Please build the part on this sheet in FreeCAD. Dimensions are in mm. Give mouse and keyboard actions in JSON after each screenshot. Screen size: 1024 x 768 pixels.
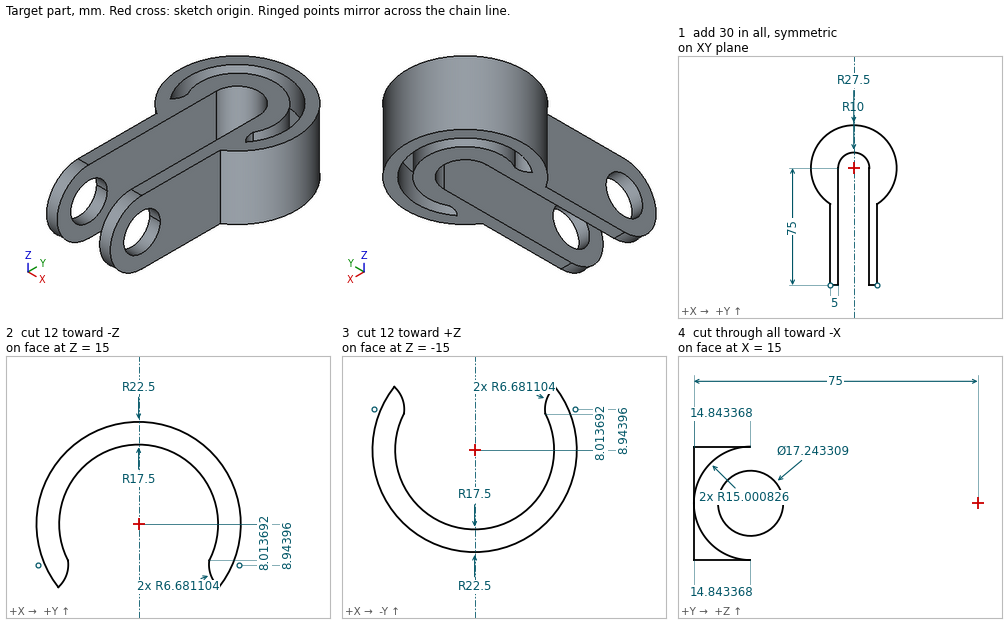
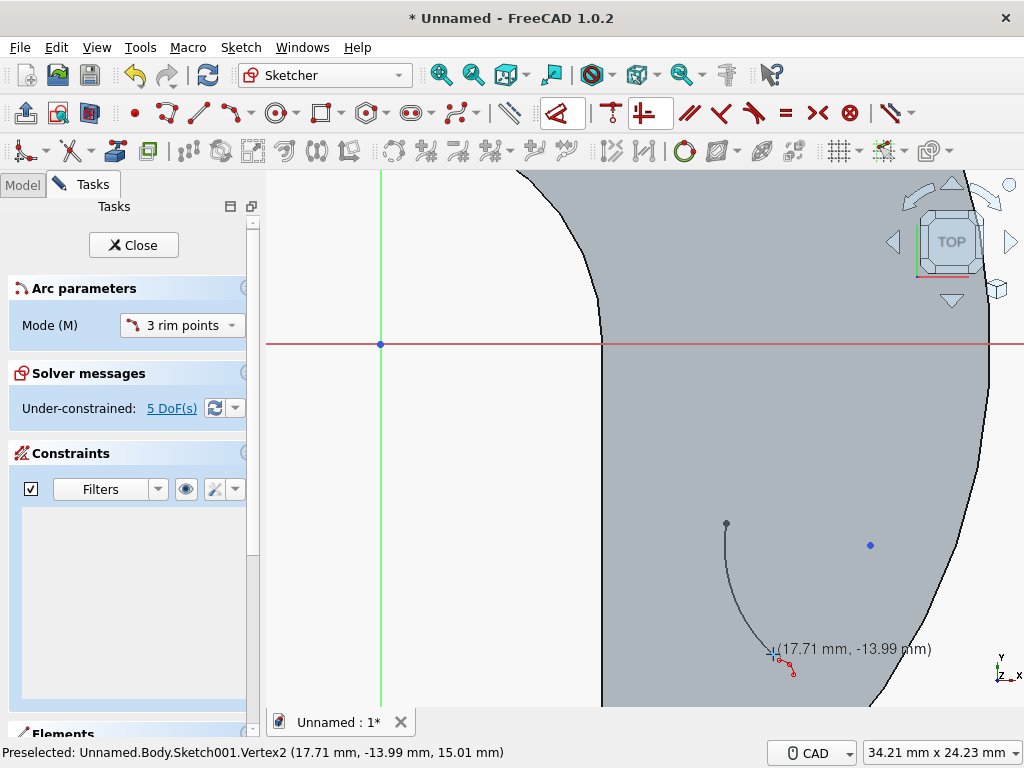
{"action": "scroll", "coordinate": [736, 593], "scroll_direction": "down", "scroll_amount": 4}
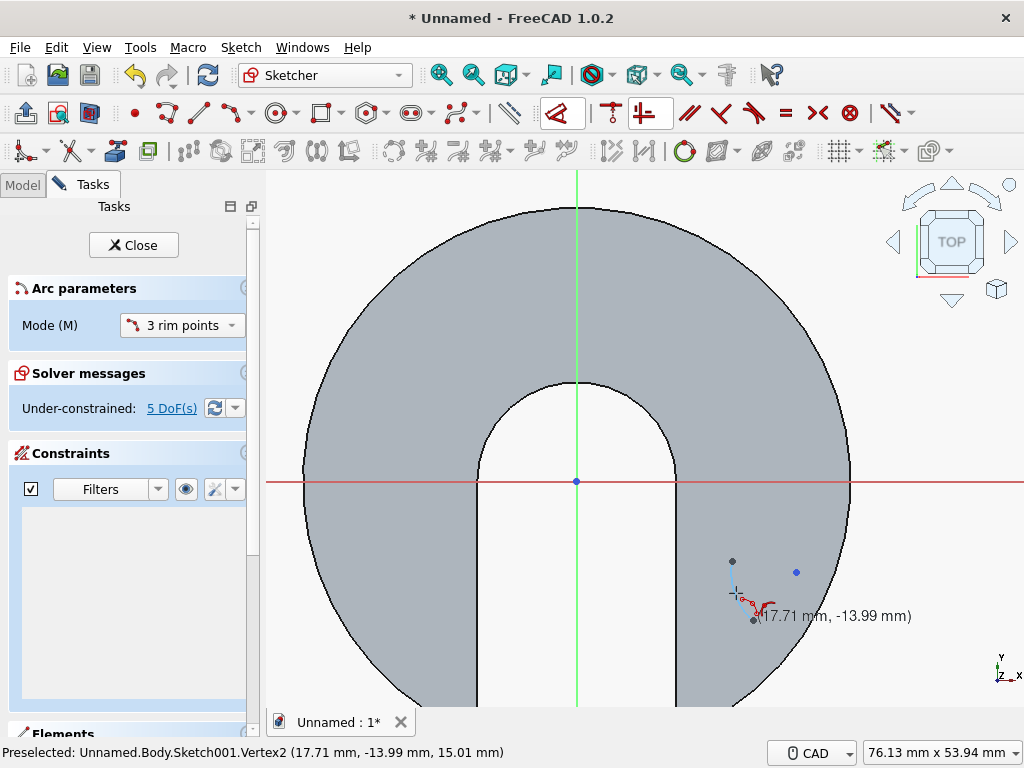
{"action": "left_click", "coordinate": [401, 620]}
{"action": "left_click", "coordinate": [674, 280]}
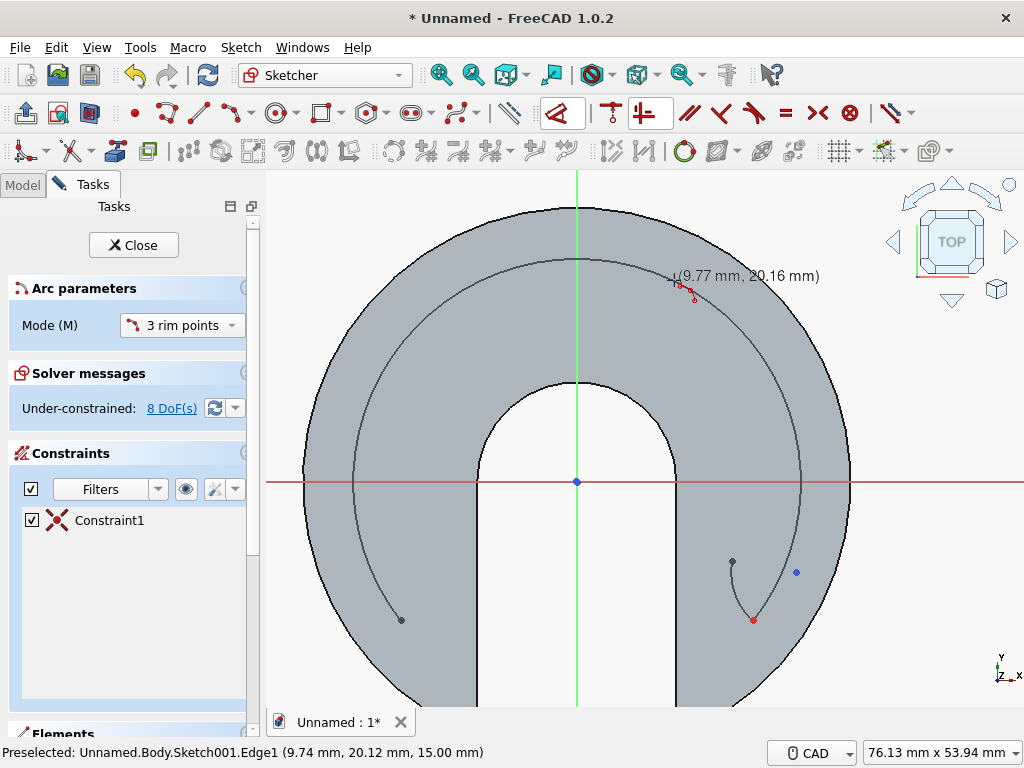
{"action": "left_click", "coordinate": [401, 621]}
{"action": "left_click", "coordinate": [422, 561]}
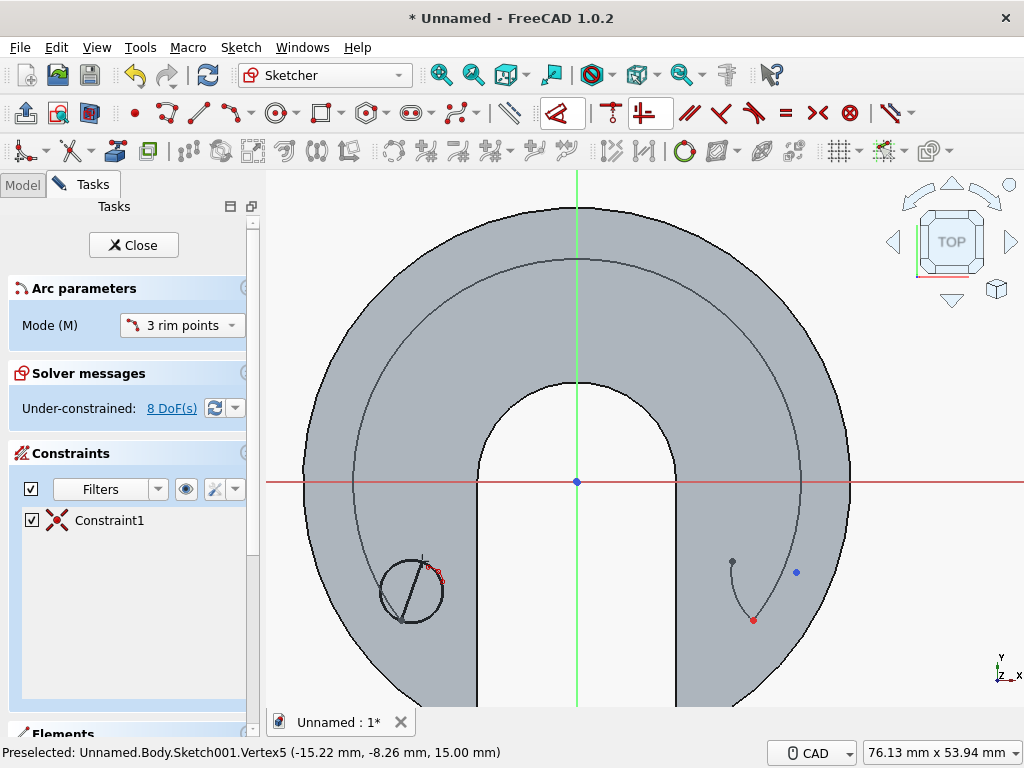
{"action": "scroll", "coordinate": [419, 593], "scroll_direction": "up", "scroll_amount": 4}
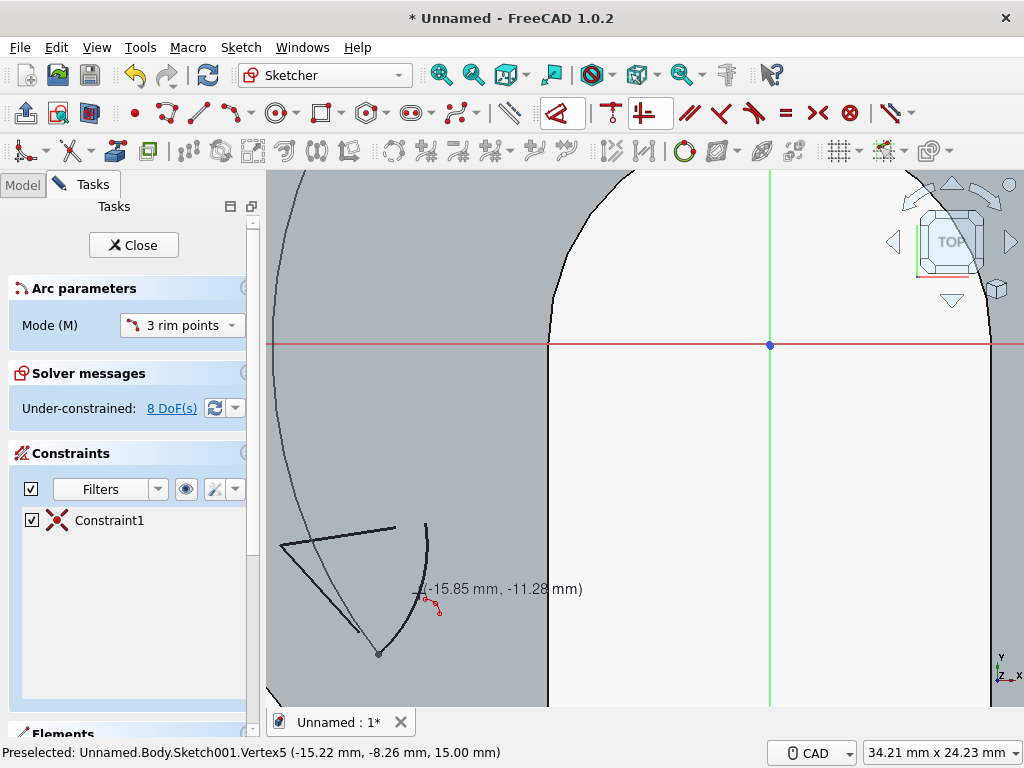
{"action": "left_click", "coordinate": [418, 593]}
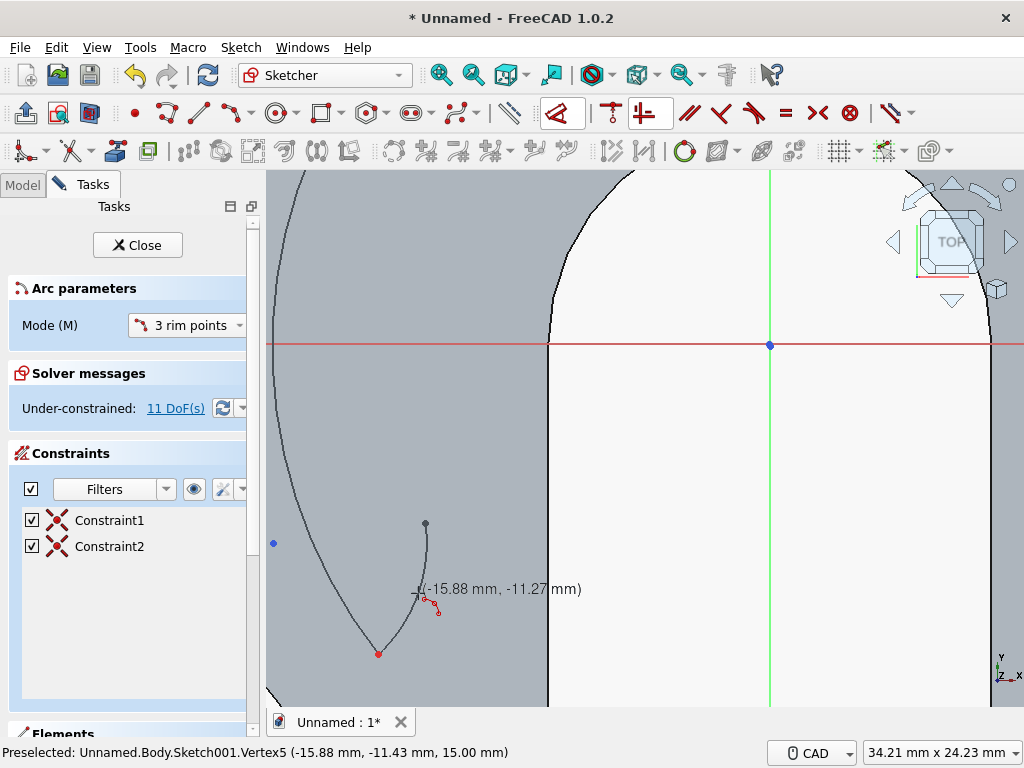
{"action": "left_click", "coordinate": [425, 523]}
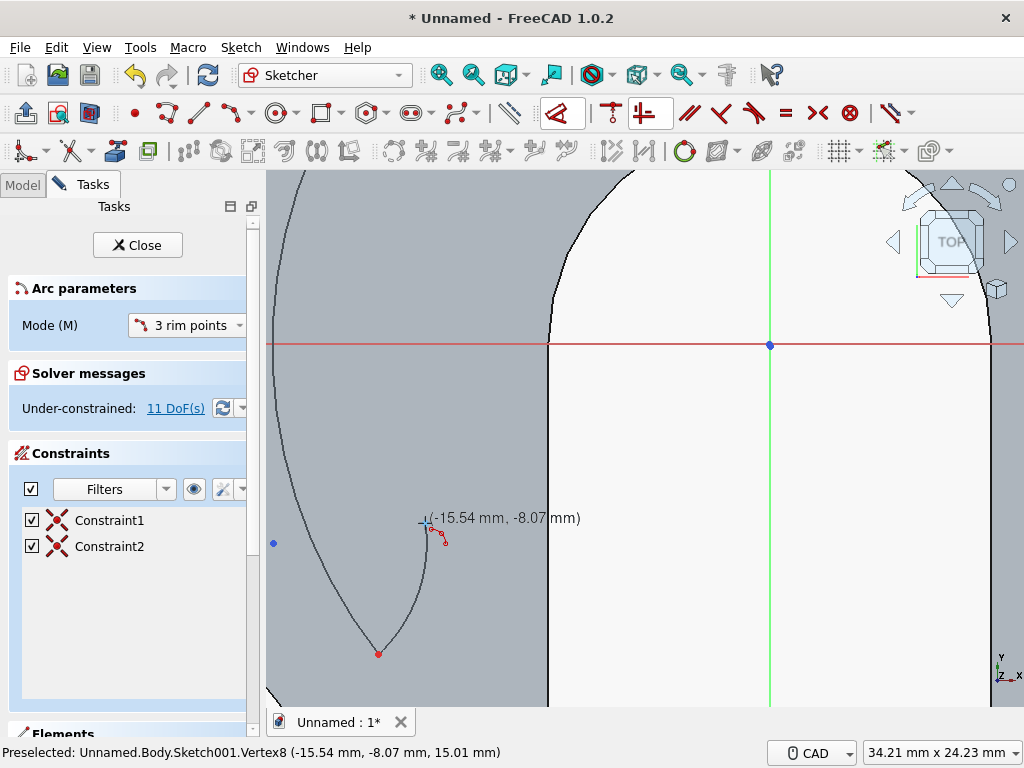
{"action": "scroll", "coordinate": [419, 593], "scroll_direction": "down", "scroll_amount": 4}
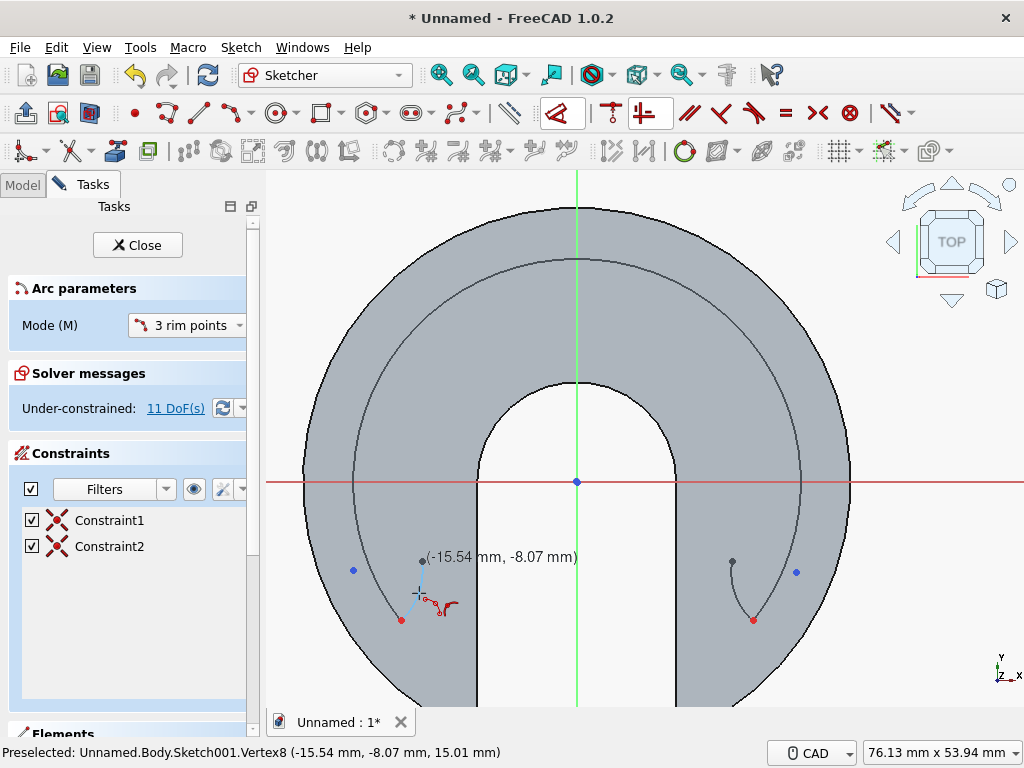
{"action": "left_click", "coordinate": [732, 562]}
{"action": "left_click", "coordinate": [646, 322]}
{"action": "key", "text": "Escape"}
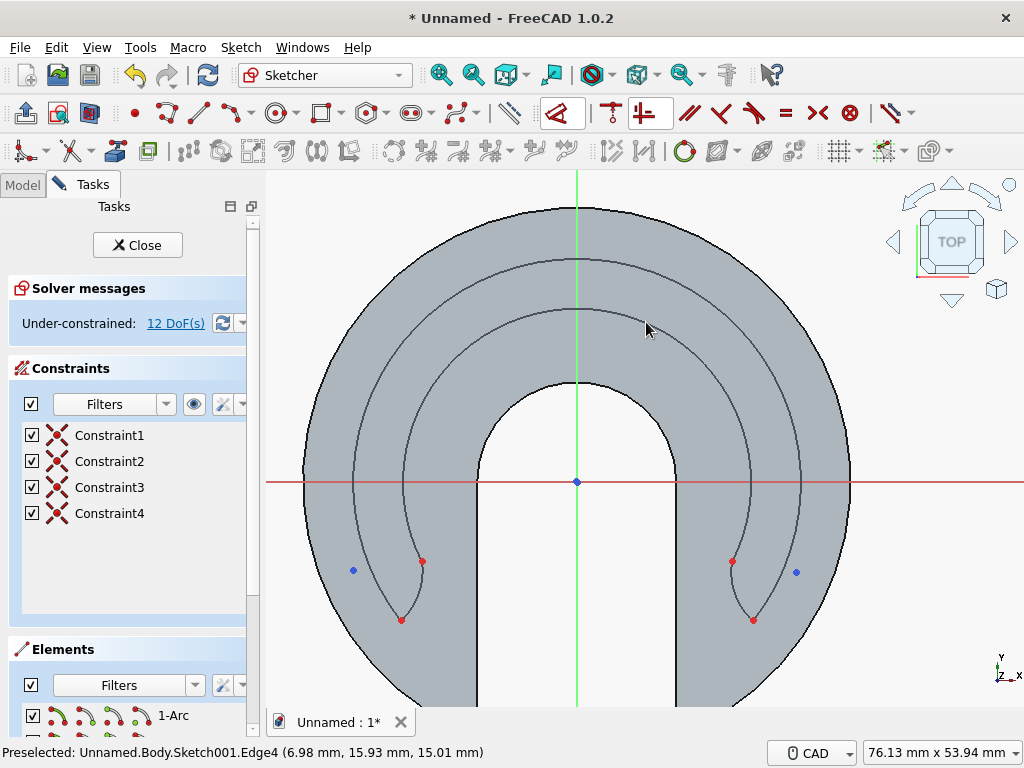
{"action": "left_click", "coordinate": [752, 343]}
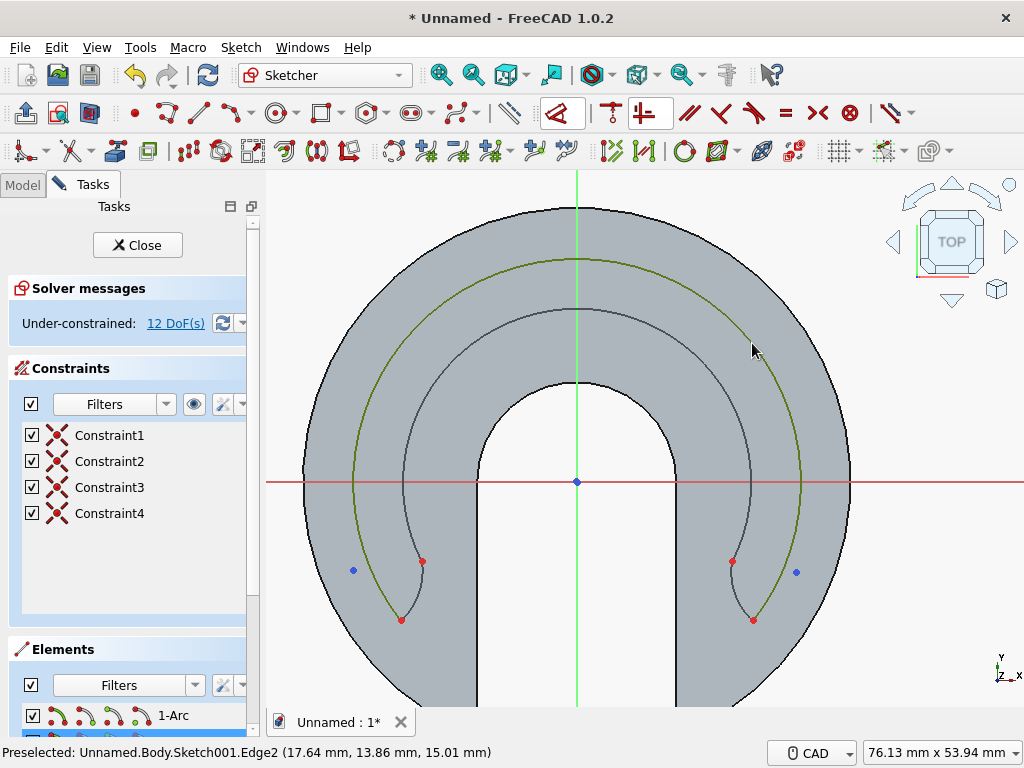
{"action": "left_click", "coordinate": [704, 364]}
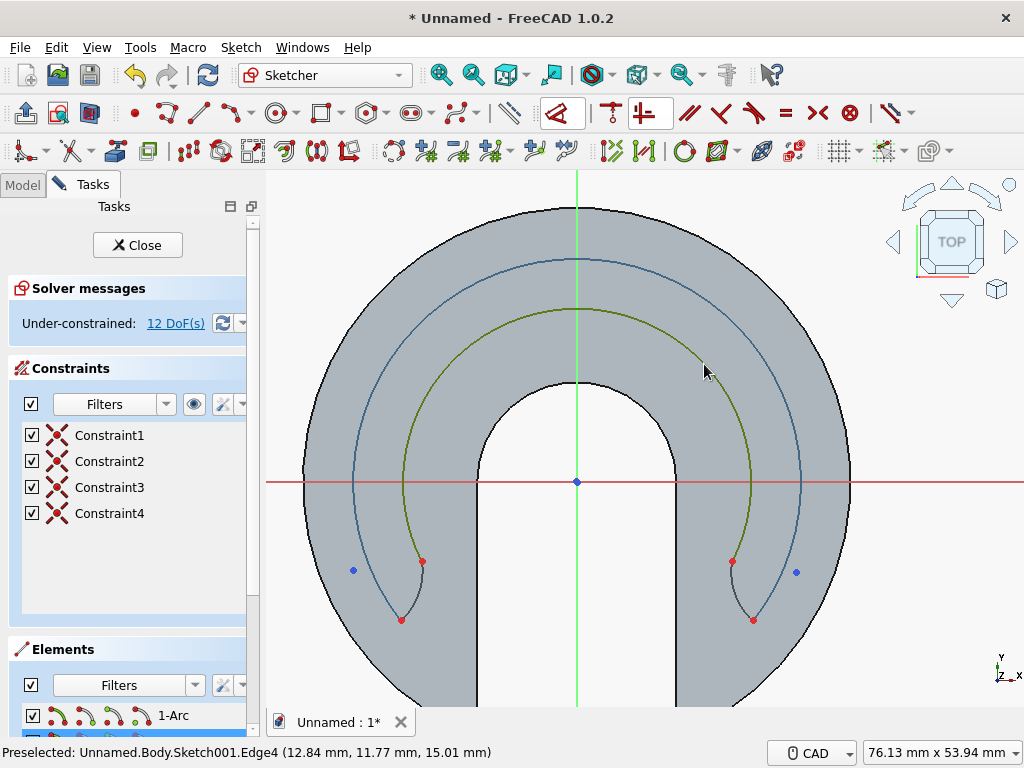
{"action": "key", "text": "c"}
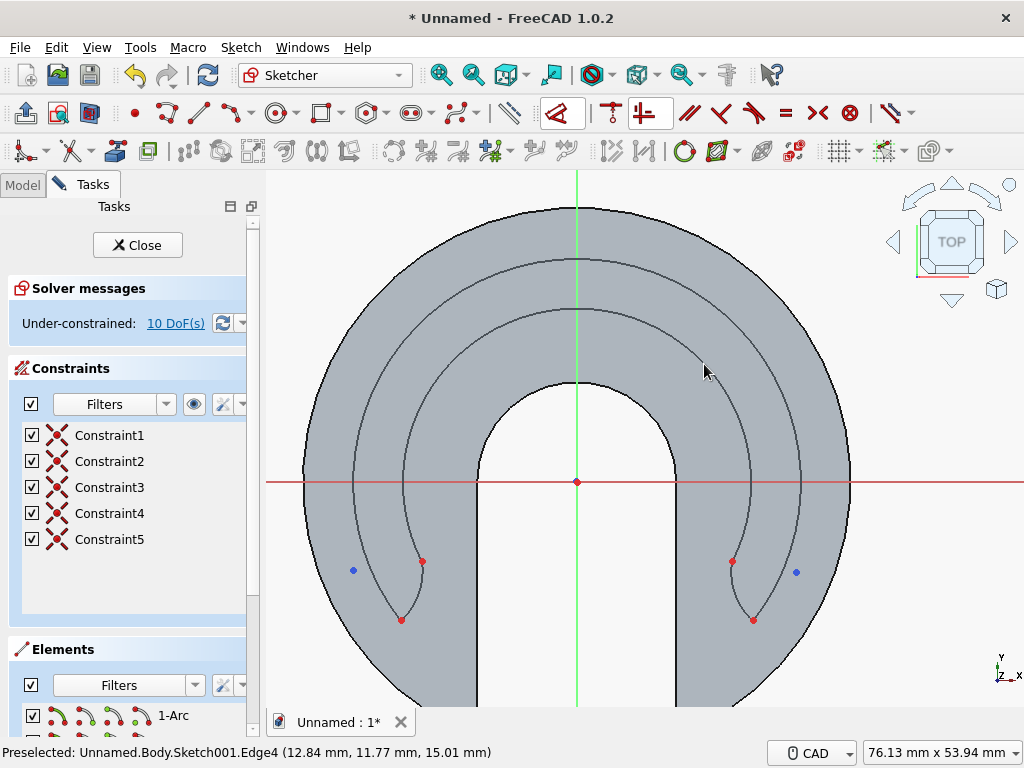
{"action": "left_click_drag", "start_coordinate": [567, 472], "coordinate": [587, 493]}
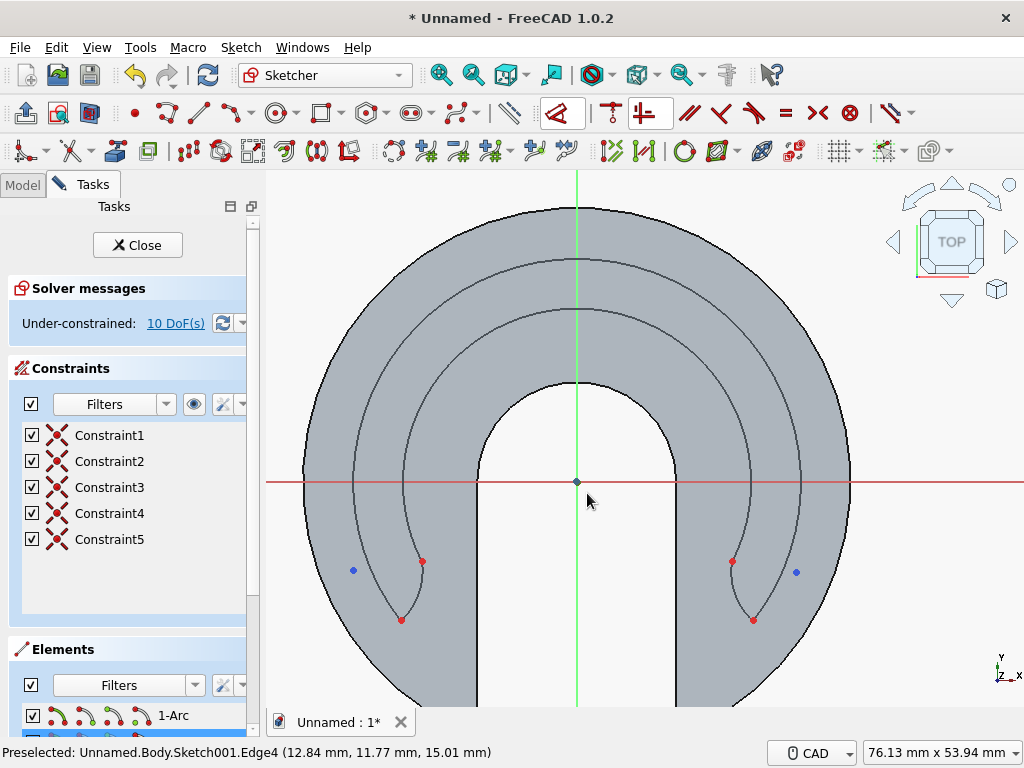
{"action": "left_click", "coordinate": [612, 114]}